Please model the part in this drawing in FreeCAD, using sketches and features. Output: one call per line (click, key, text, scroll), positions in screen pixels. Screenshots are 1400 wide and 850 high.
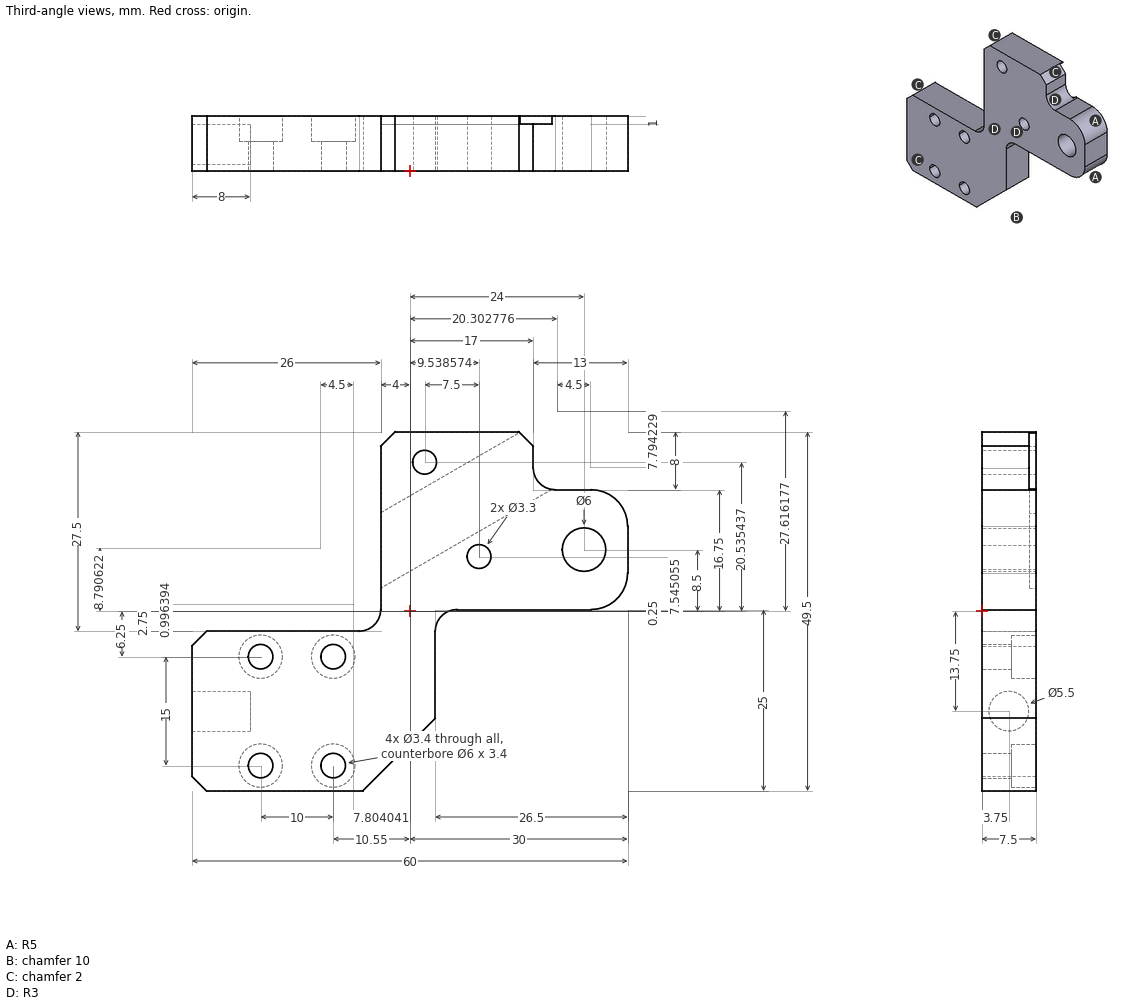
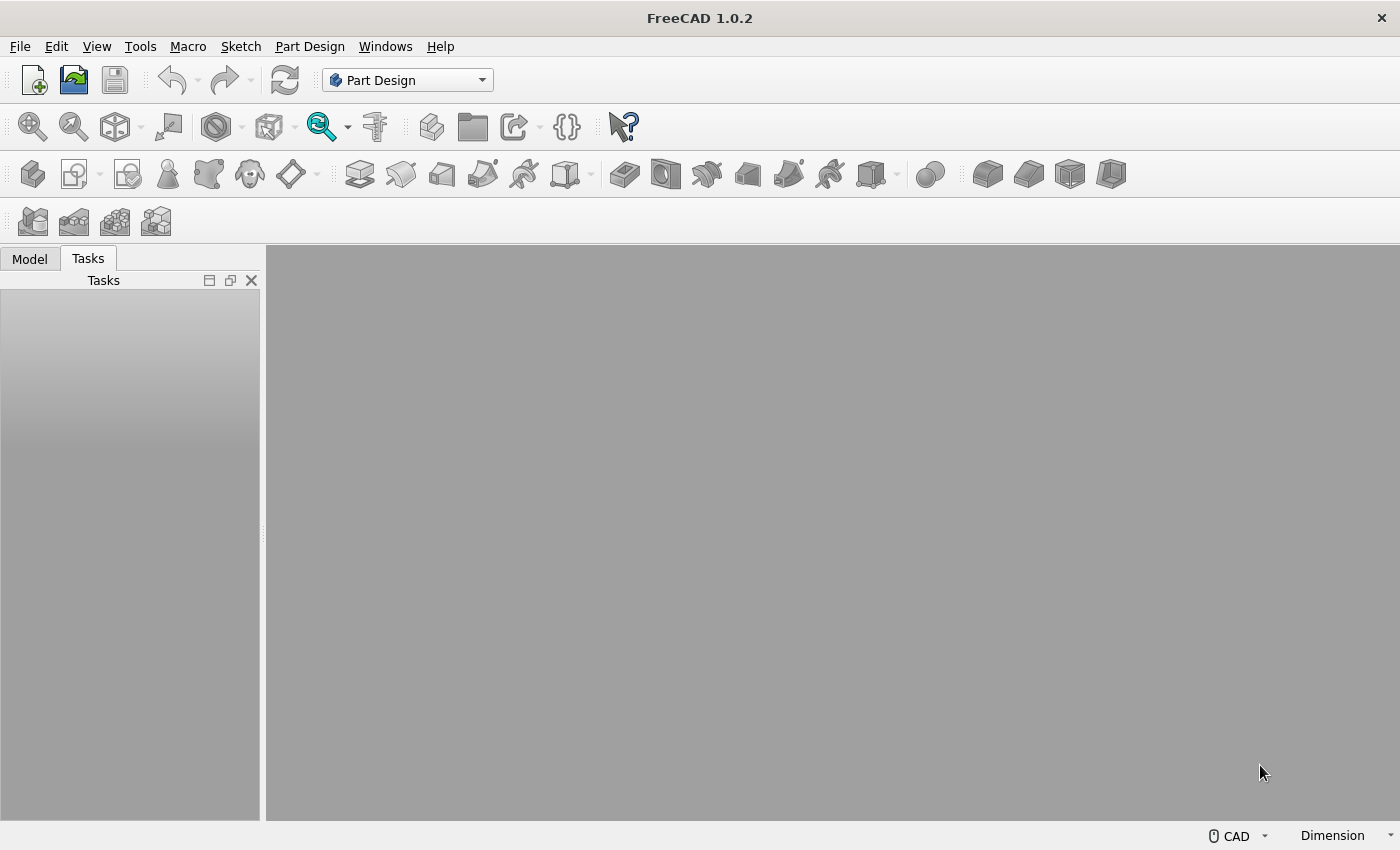
click(33, 80)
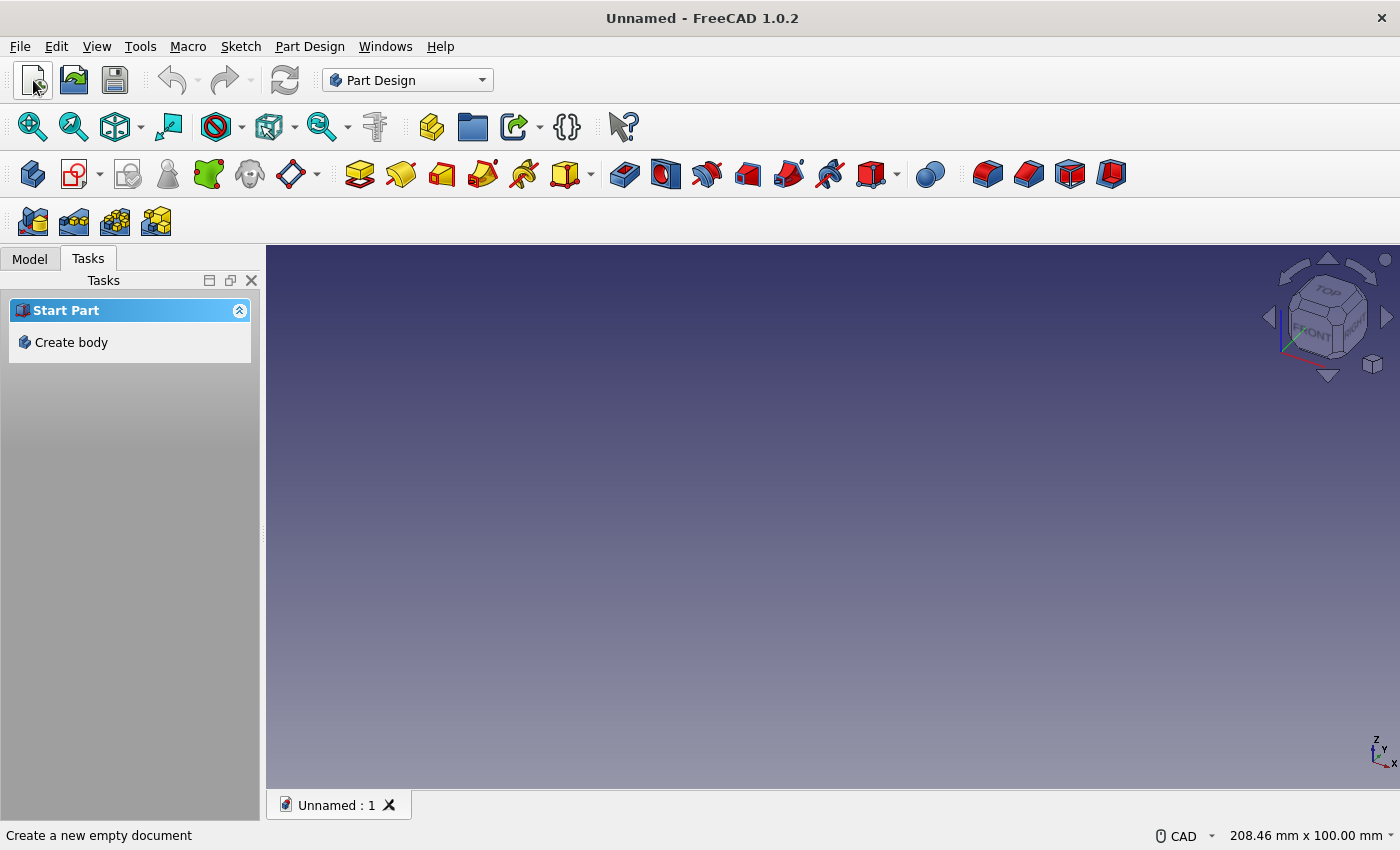
click(74, 174)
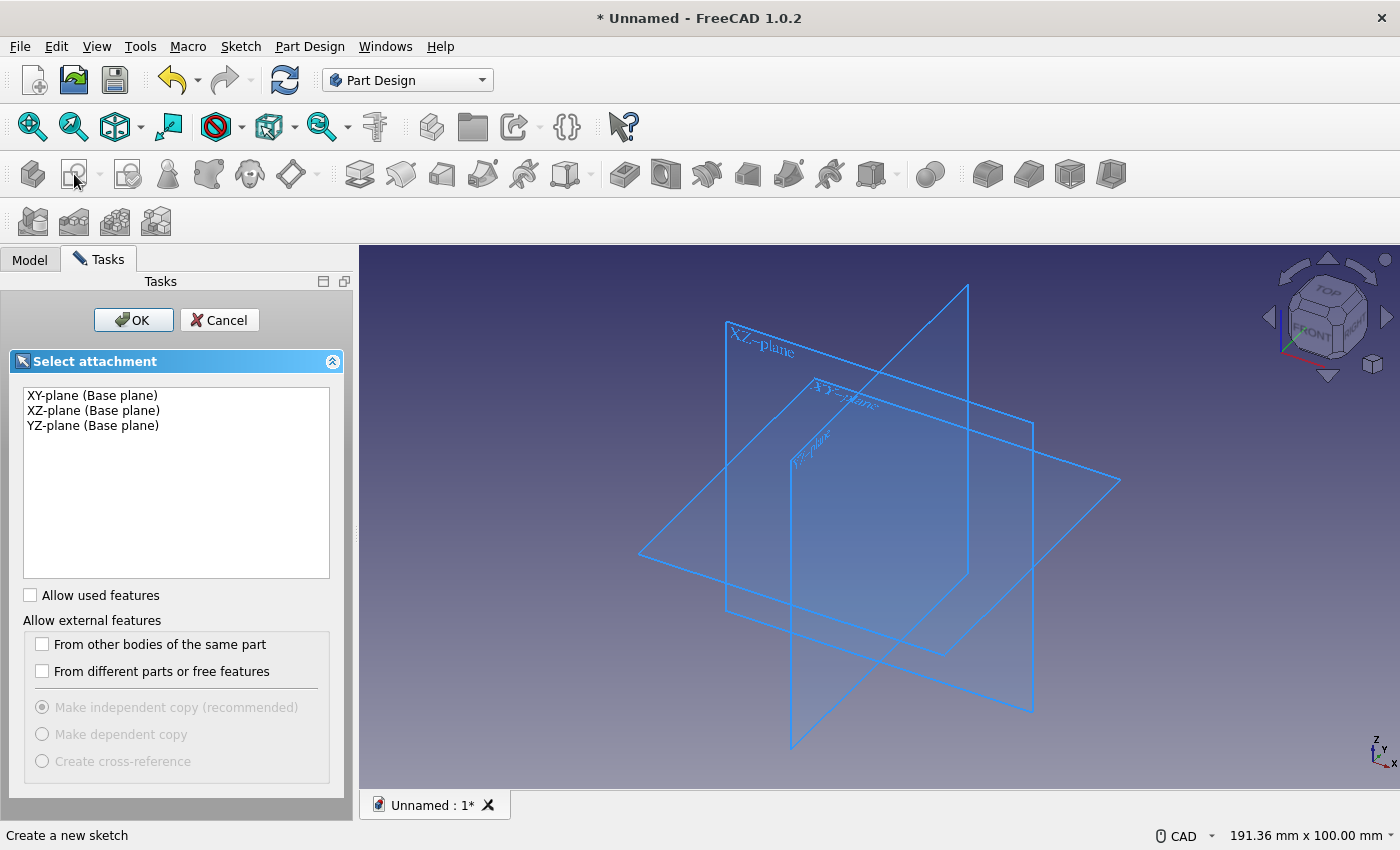
click(84, 410)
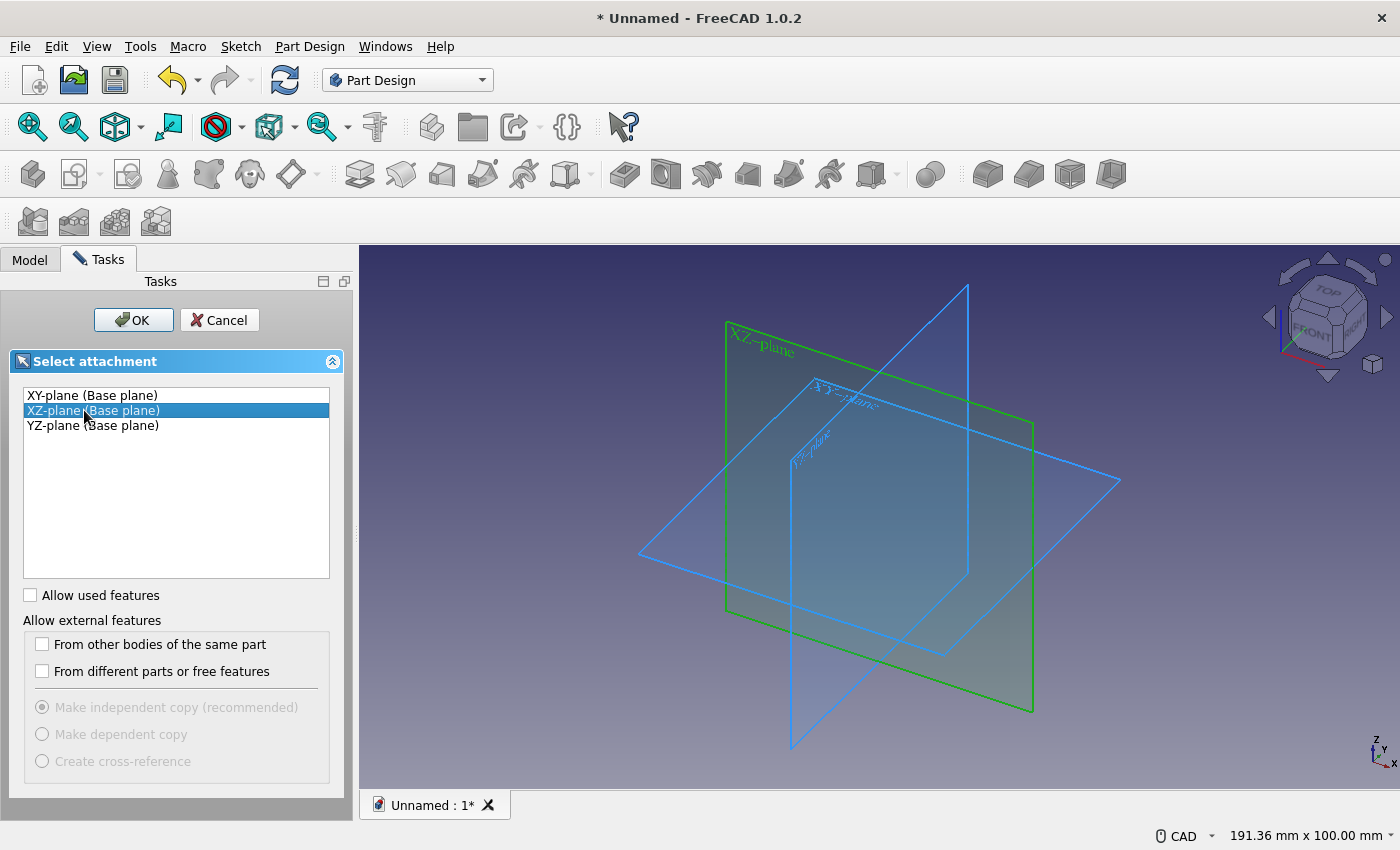
click(134, 320)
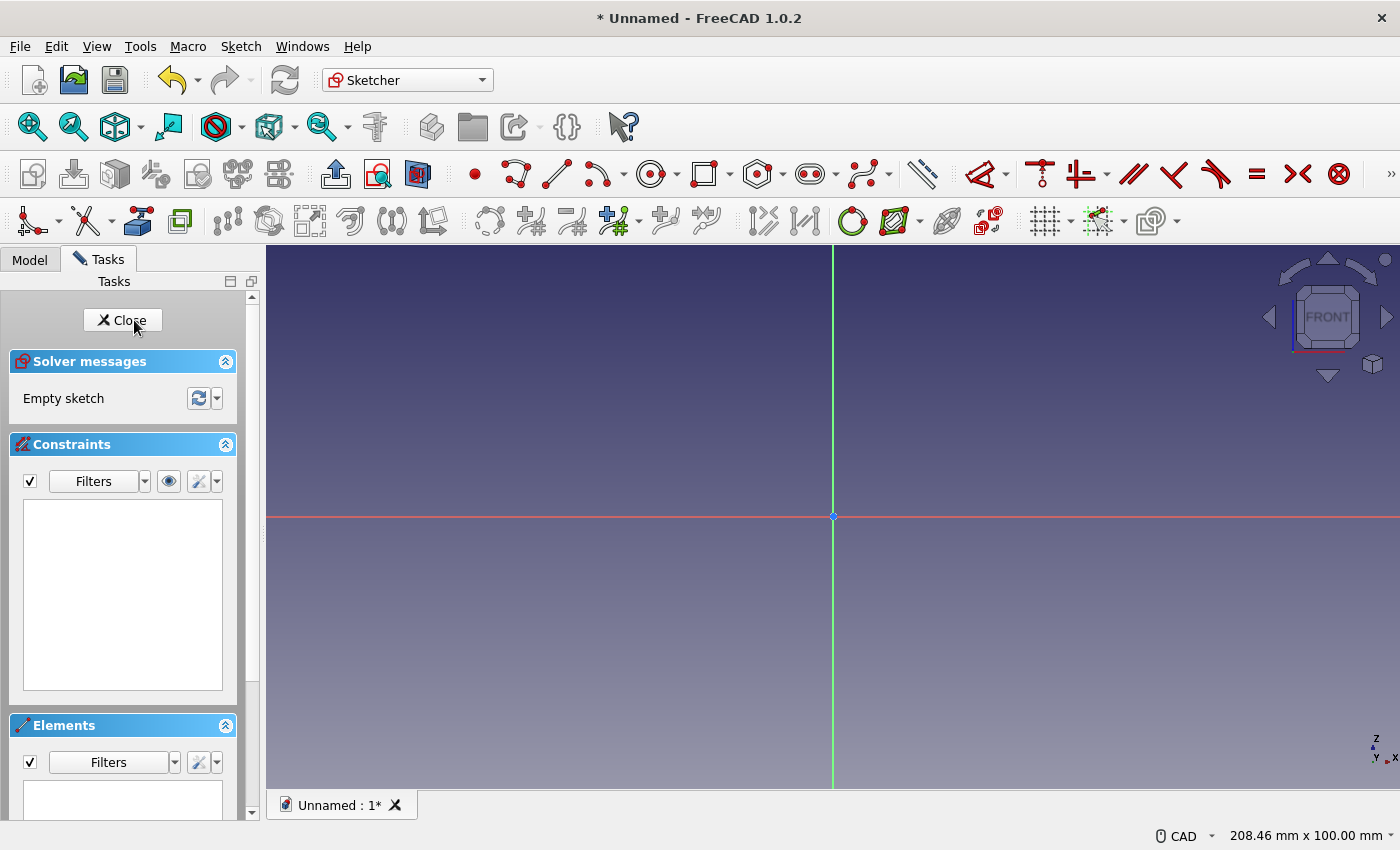
key(g)
key(v)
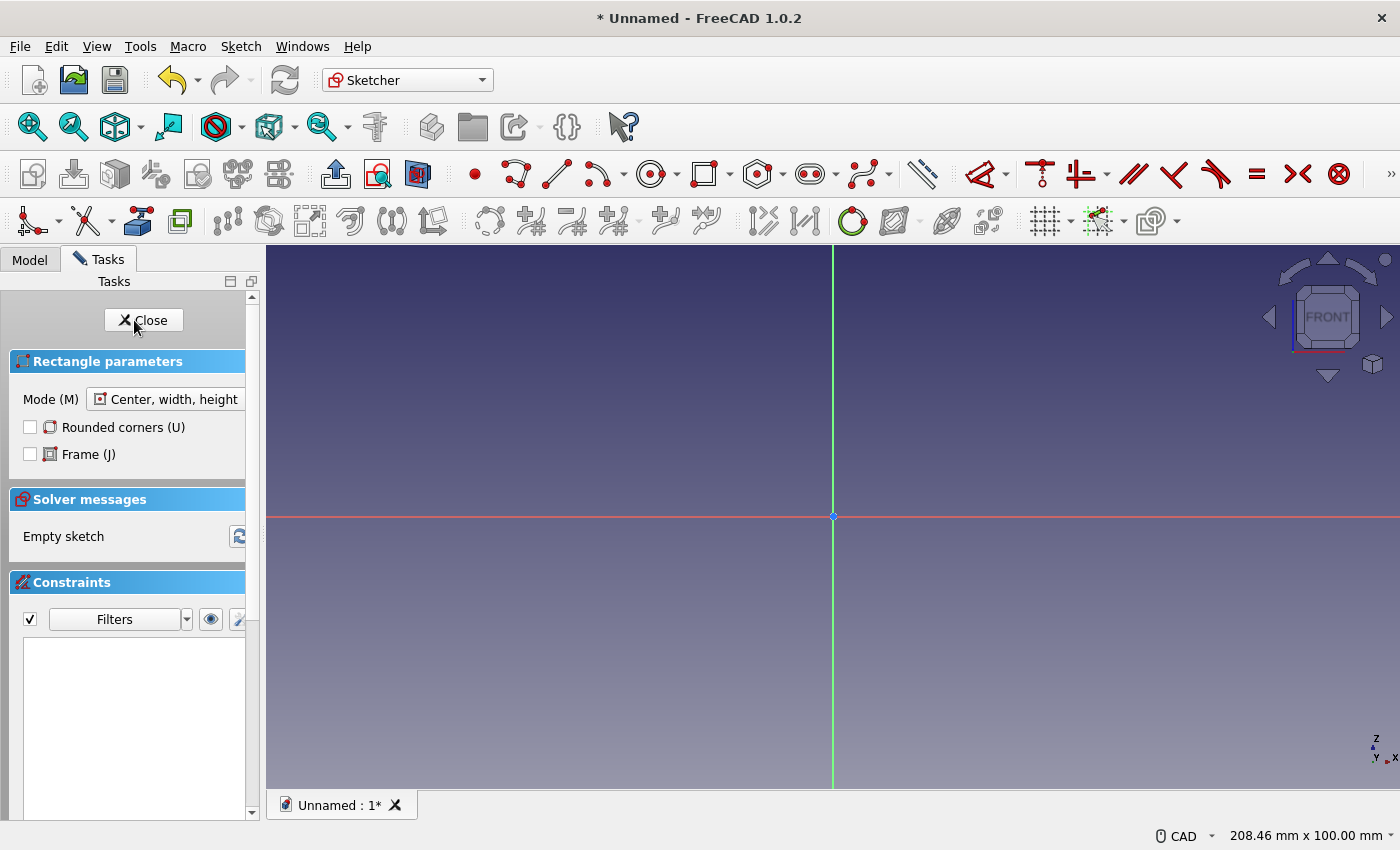
click(833, 517)
move(996, 382)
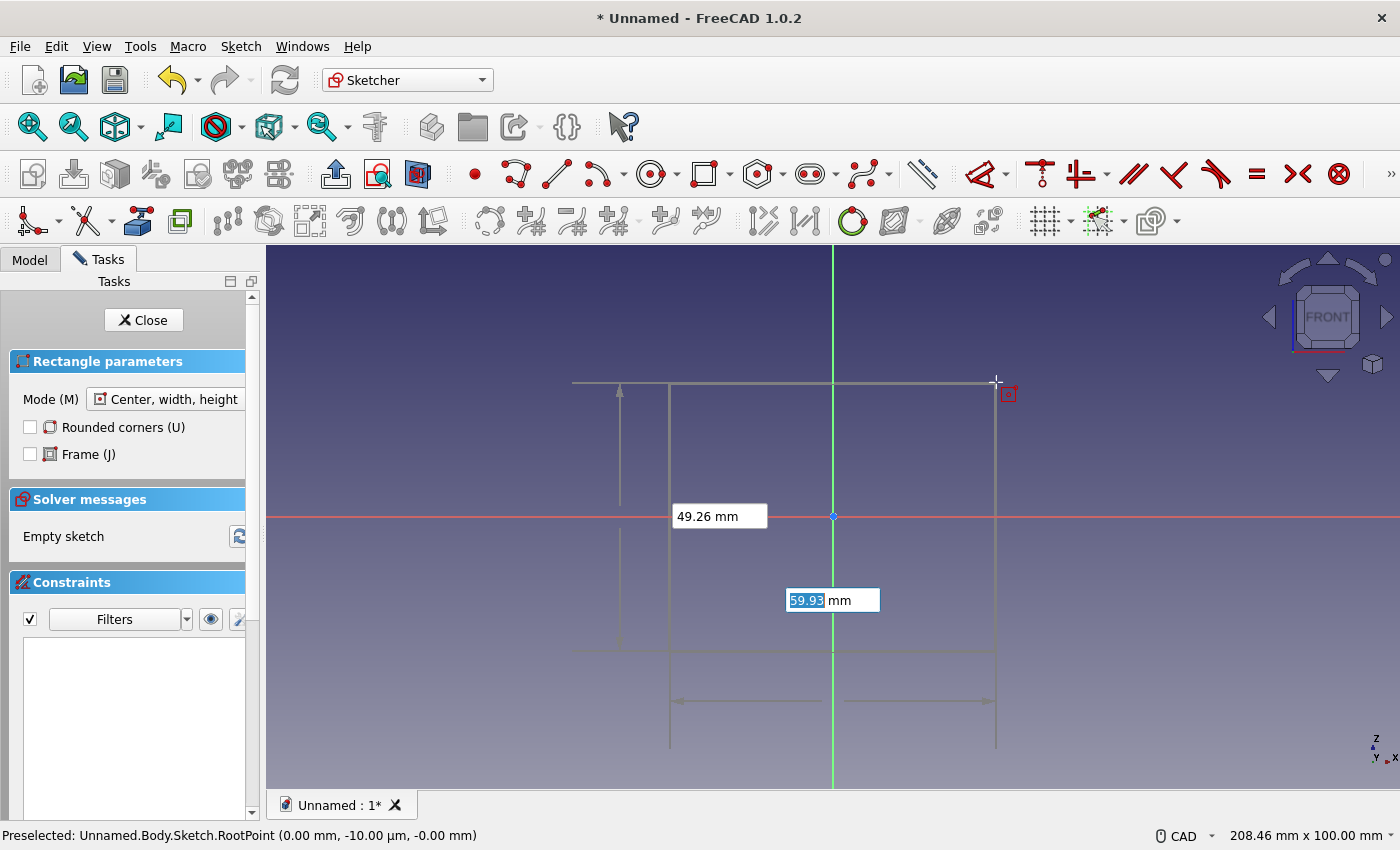
text(60)
key(Tab)
text(49.5)
key(Return)
key(Escape)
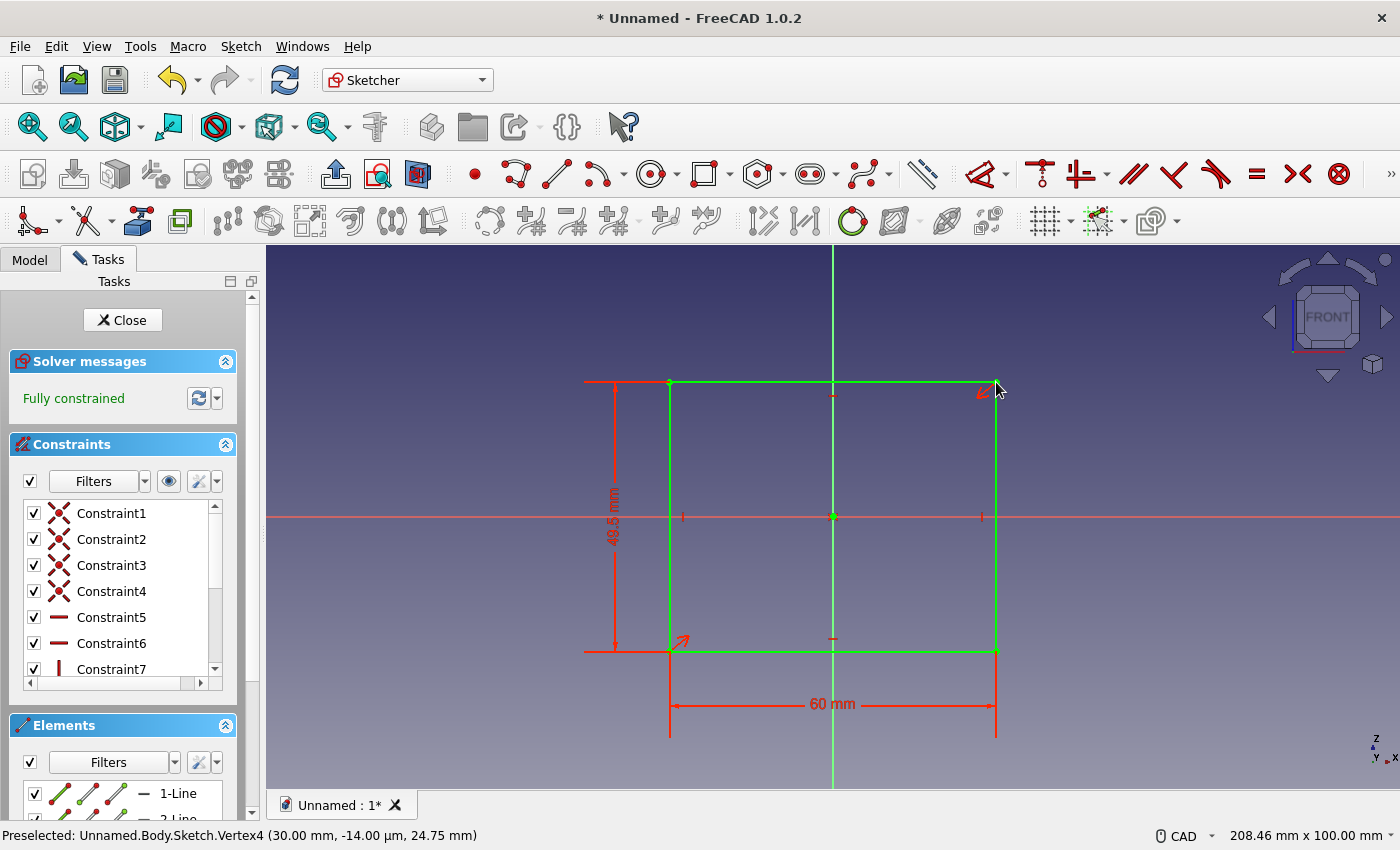
click(123, 320)